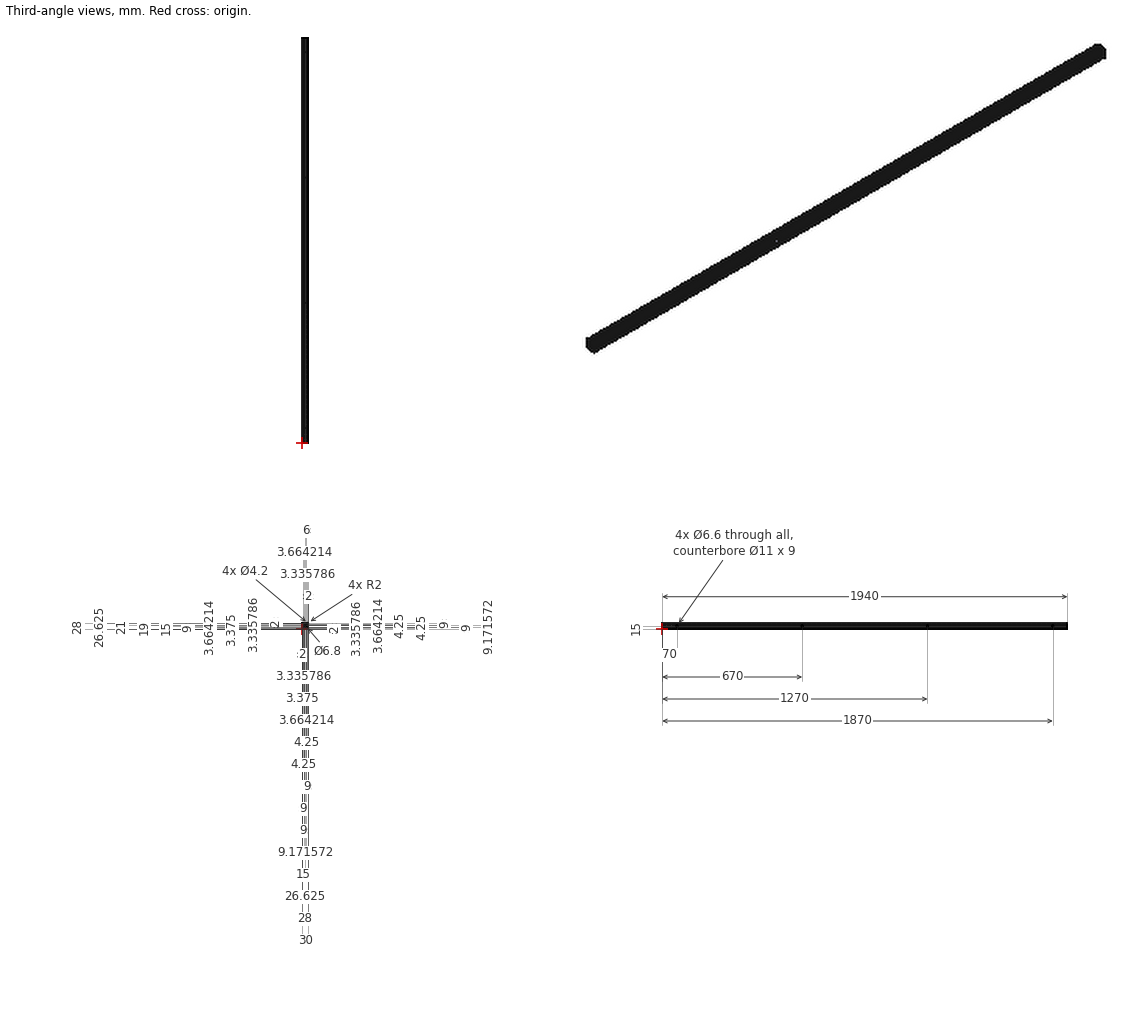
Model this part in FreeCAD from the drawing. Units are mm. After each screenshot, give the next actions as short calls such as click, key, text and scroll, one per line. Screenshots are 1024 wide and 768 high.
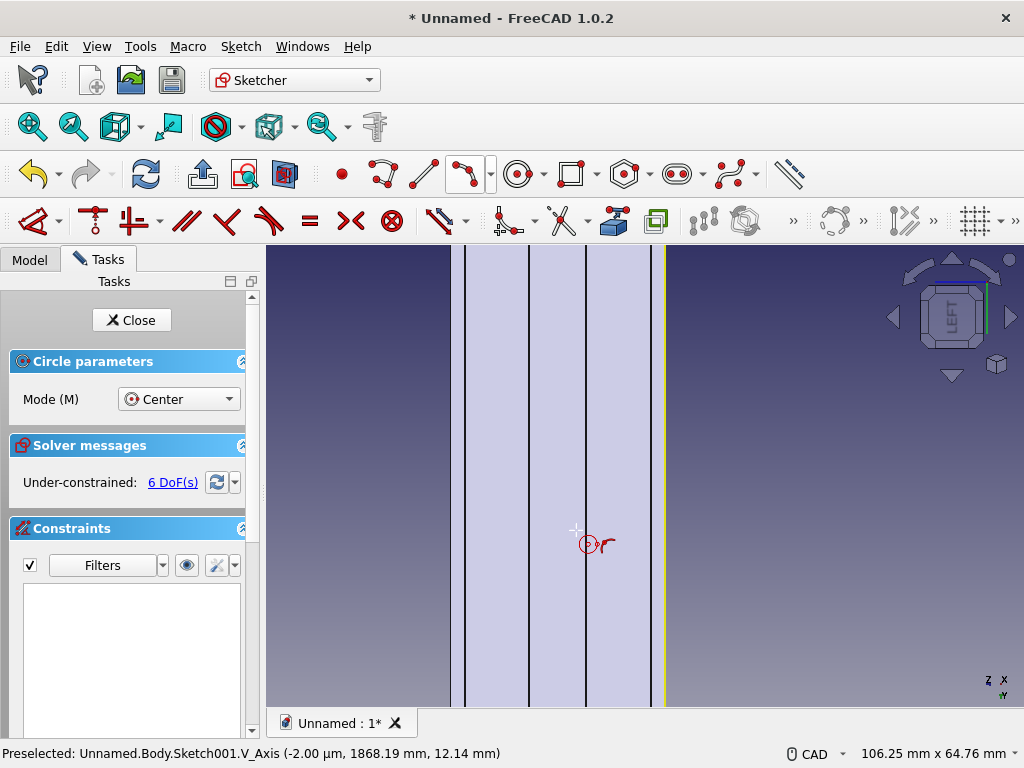
scroll(576, 476, down, 15)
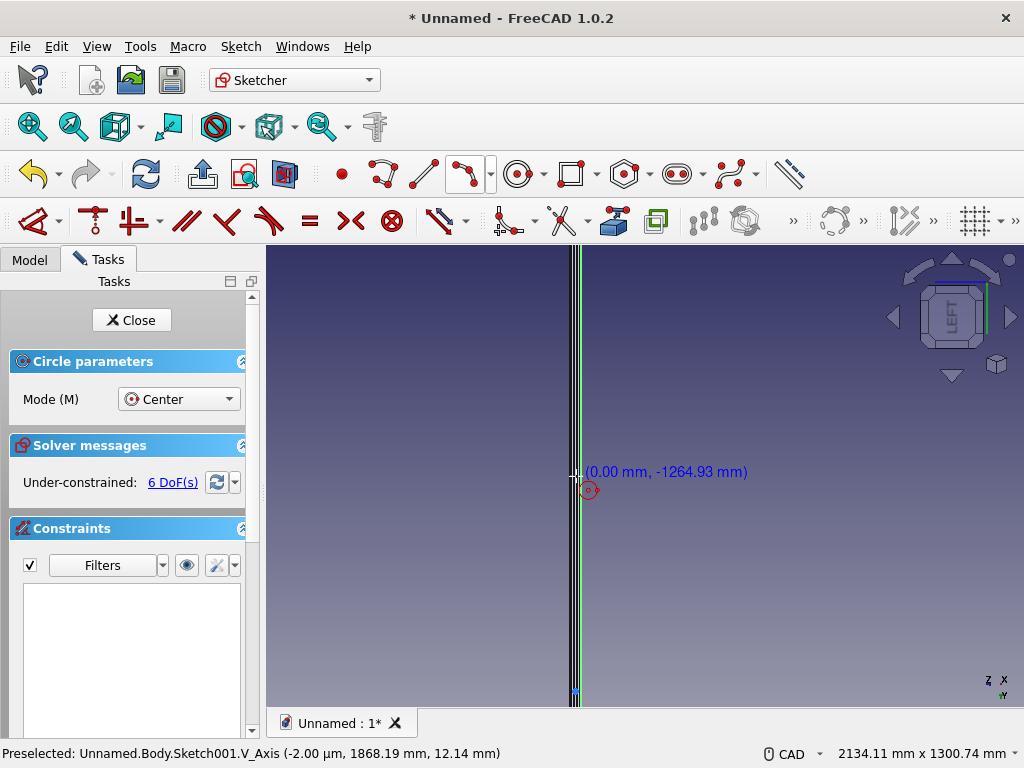
scroll(576, 571, down, 4)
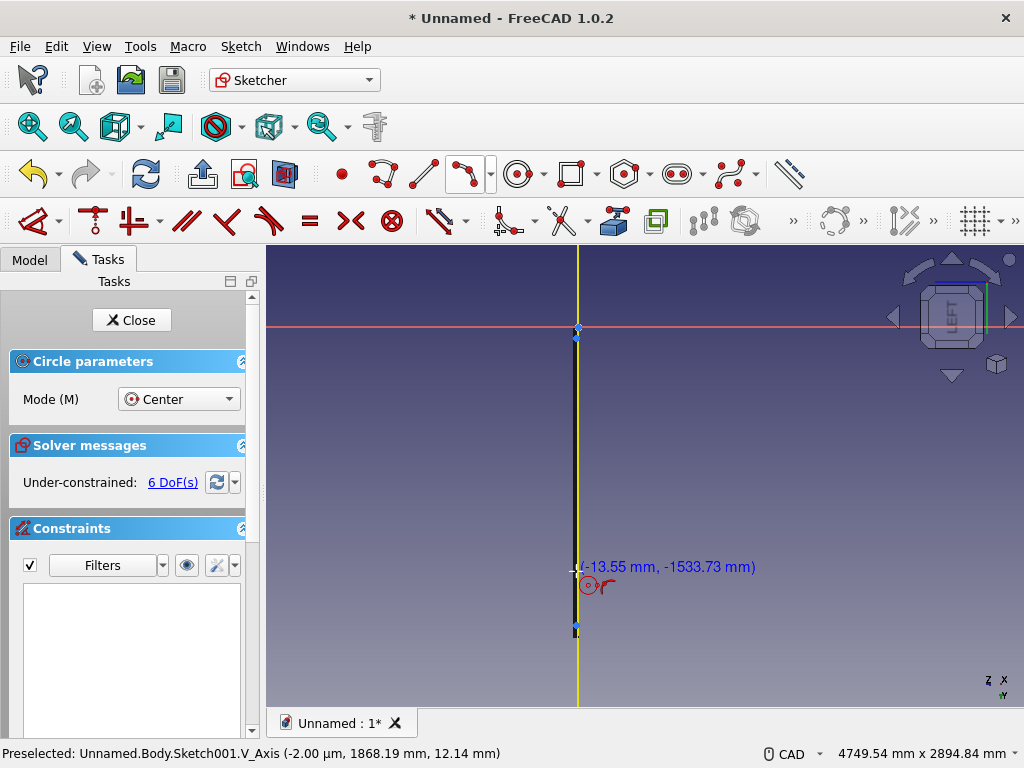
scroll(576, 530, up, 10)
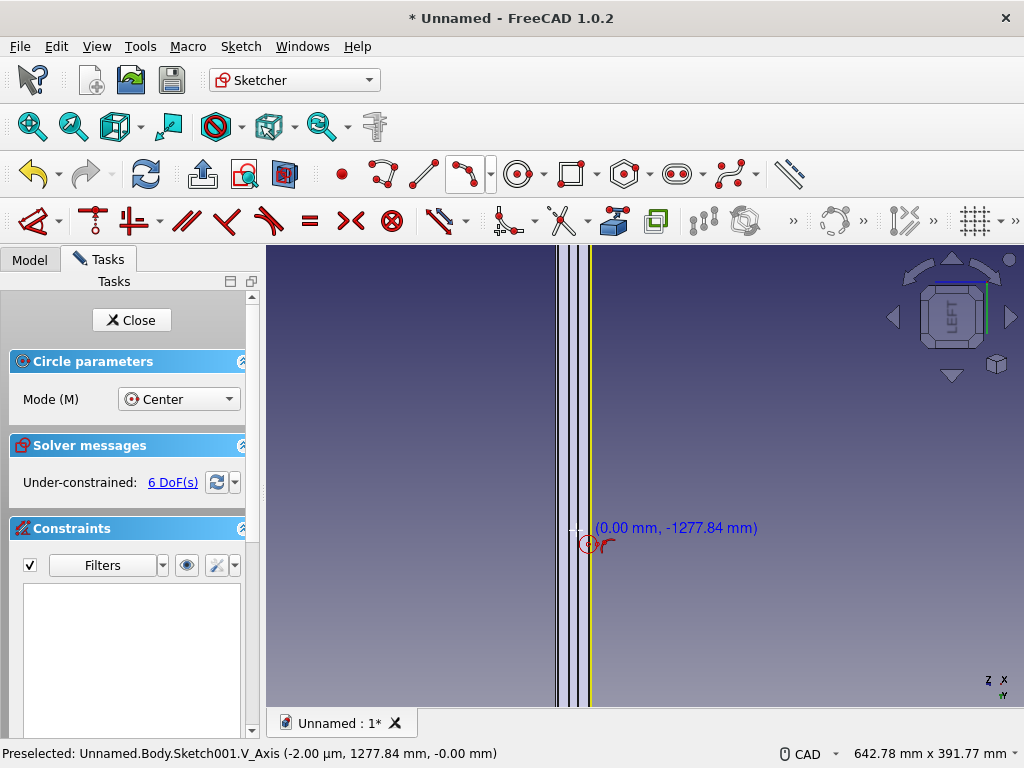
click(573, 524)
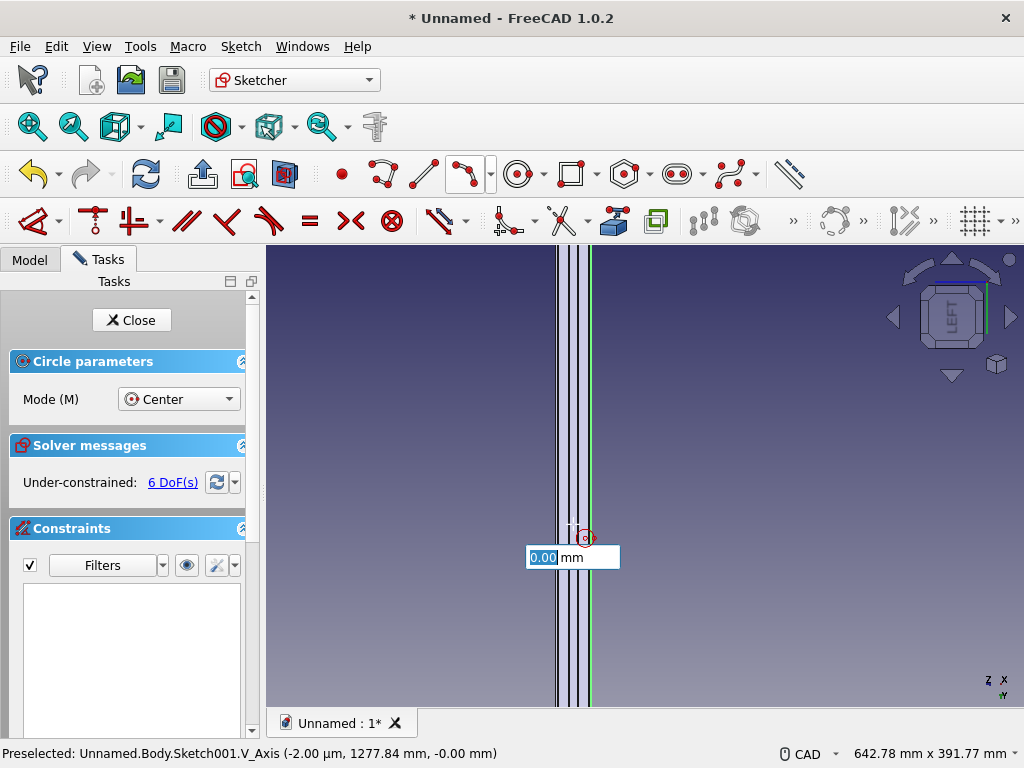
scroll(576, 521, up, 8)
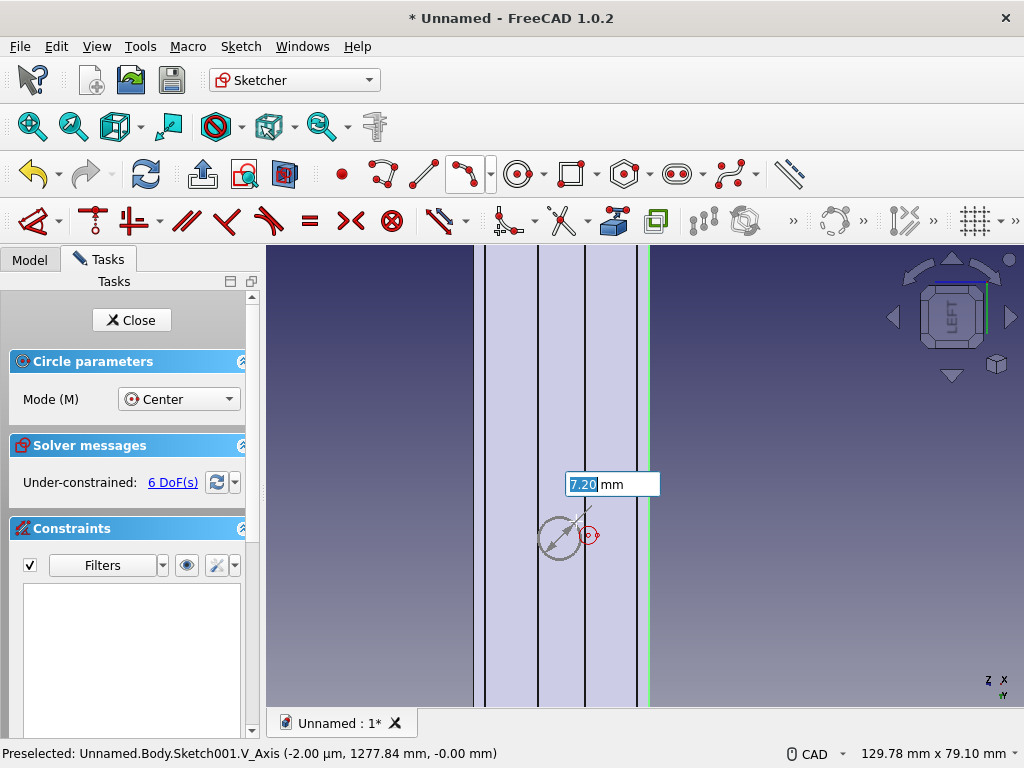
click(575, 521)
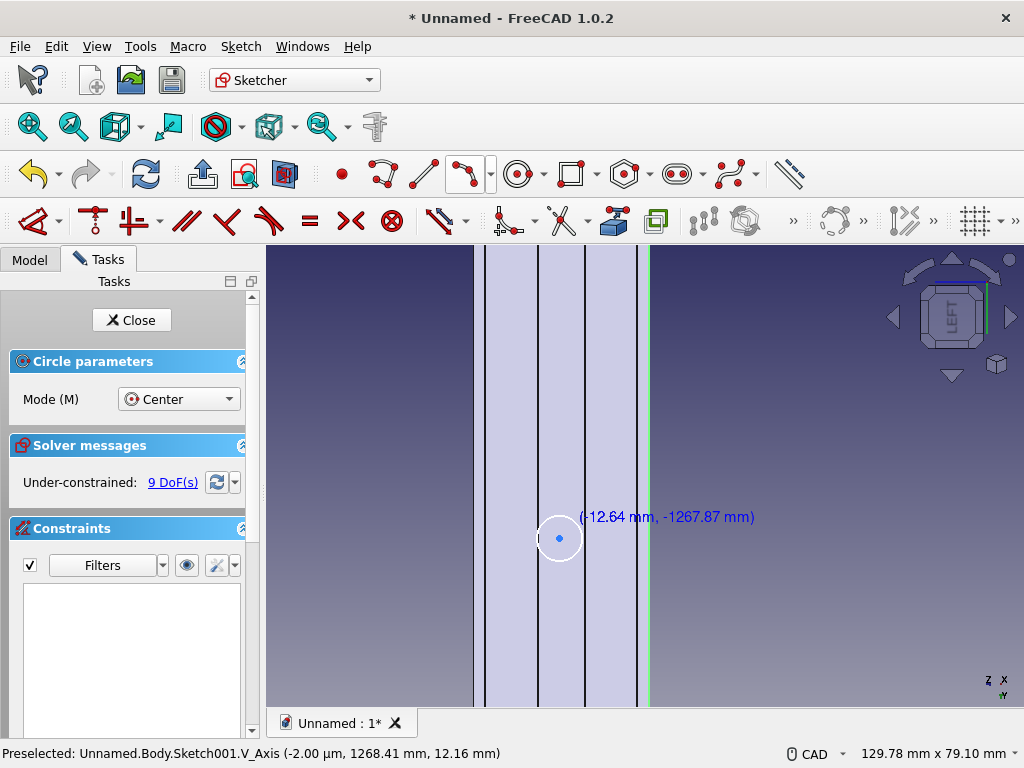
scroll(576, 529, down, 18)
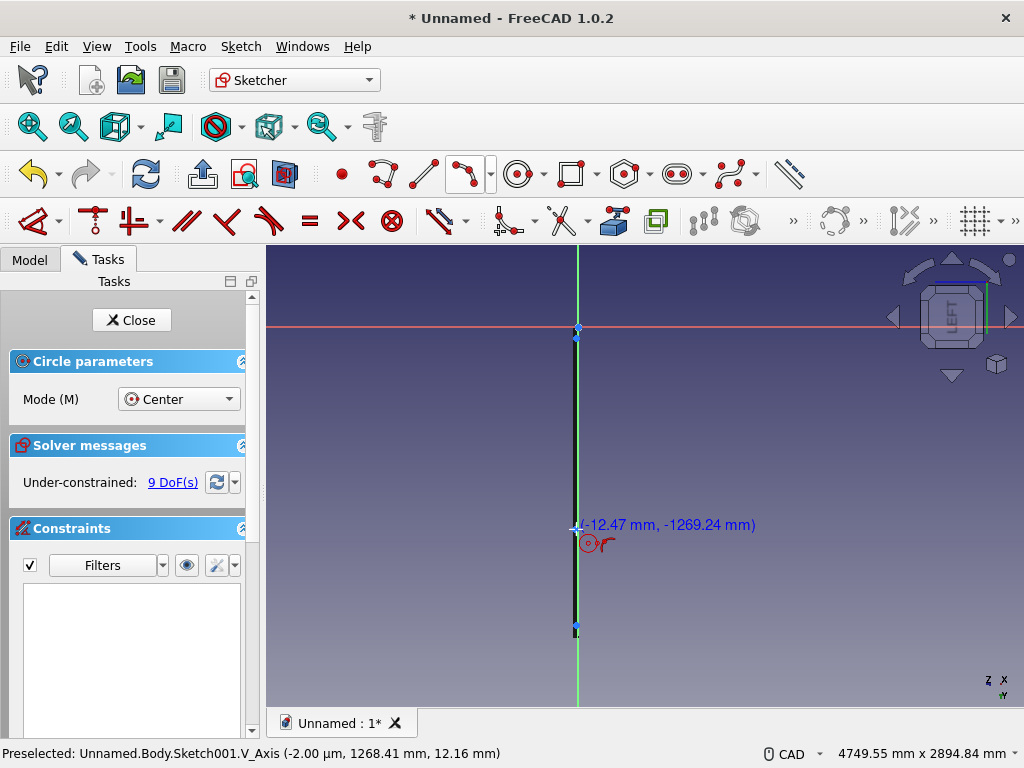
scroll(576, 434, up, 19)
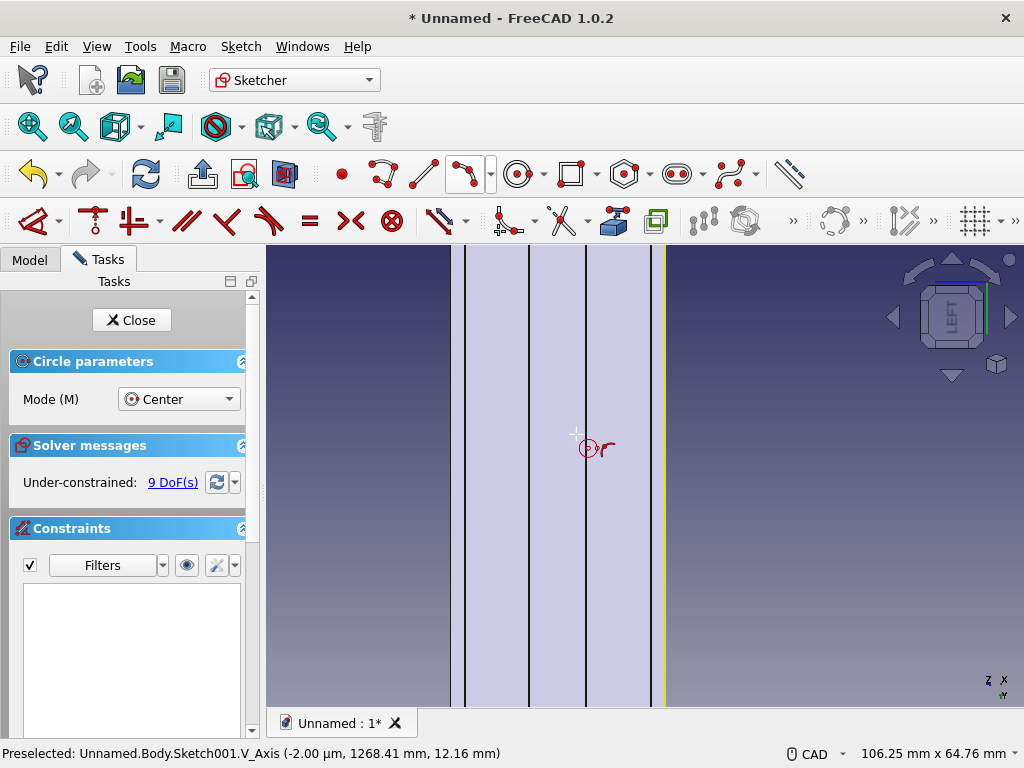
scroll(576, 476, down, 15)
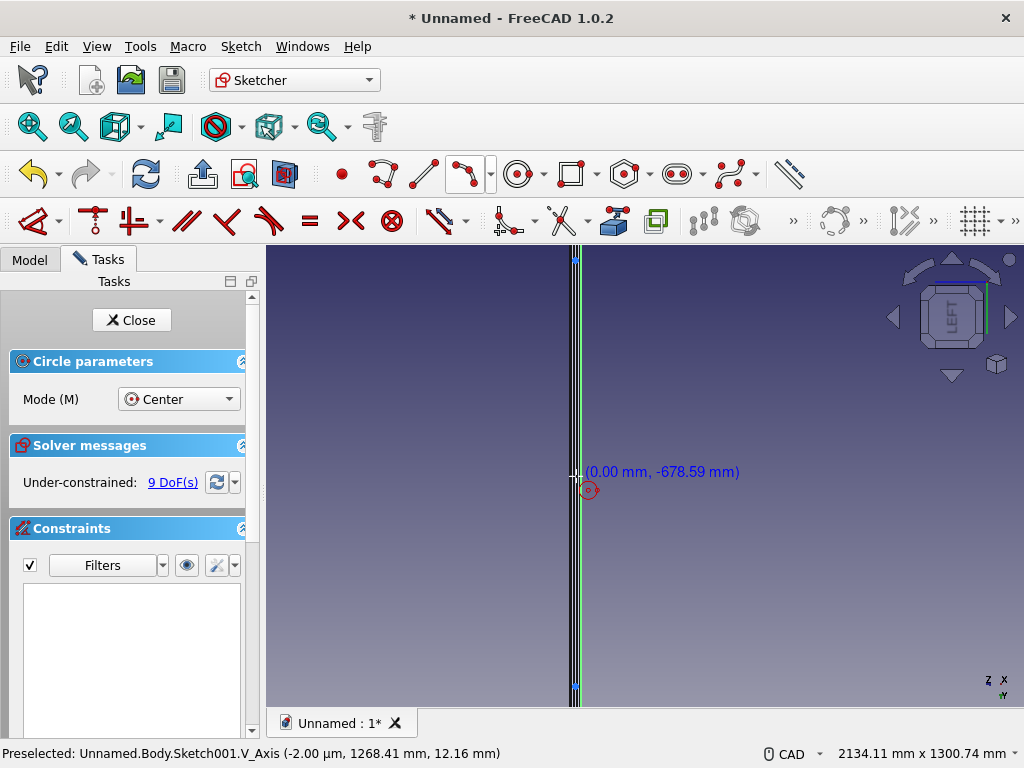
scroll(576, 401, down, 4)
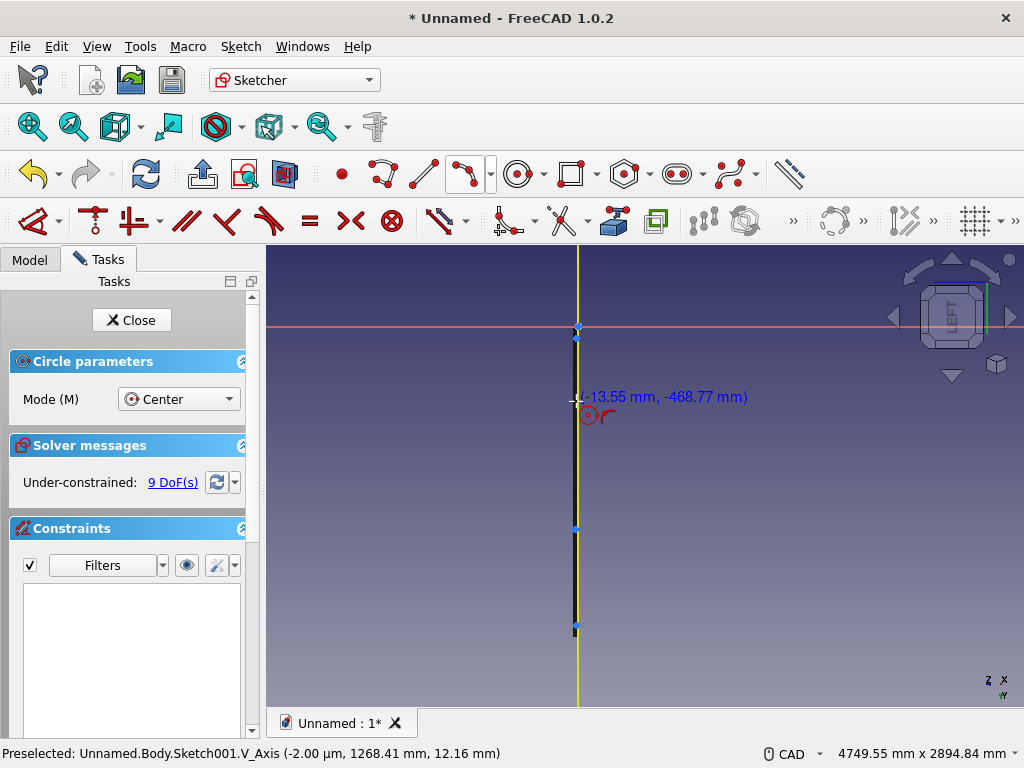
scroll(576, 434, up, 10)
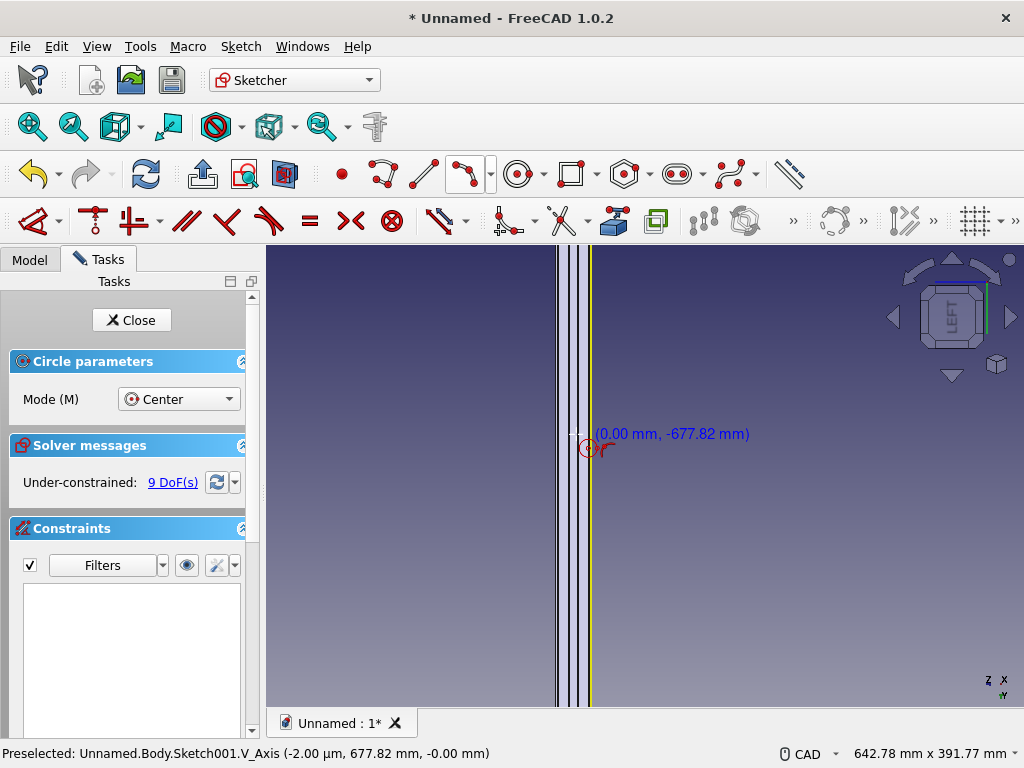
click(573, 430)